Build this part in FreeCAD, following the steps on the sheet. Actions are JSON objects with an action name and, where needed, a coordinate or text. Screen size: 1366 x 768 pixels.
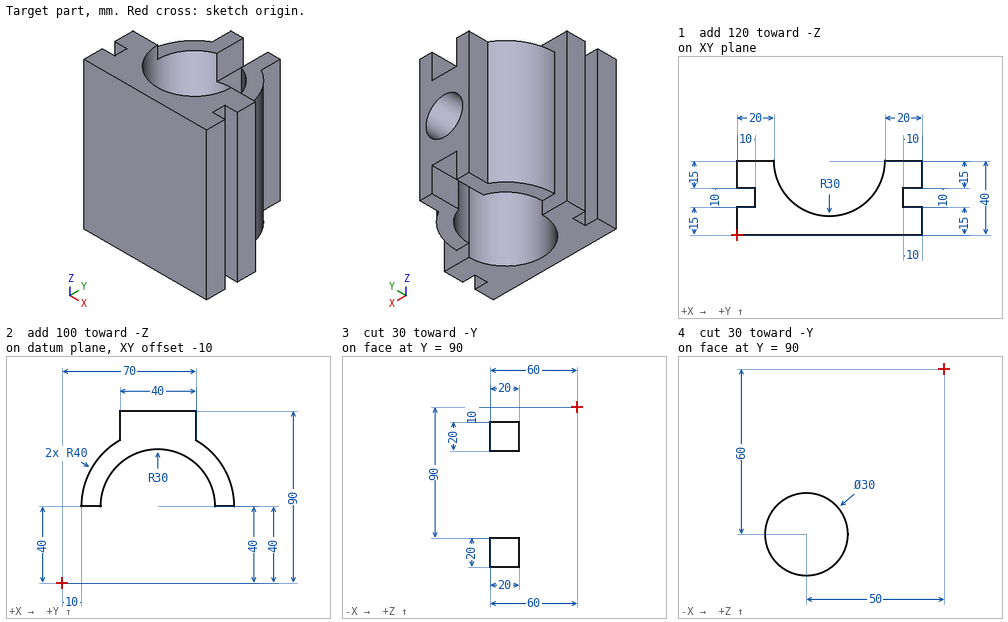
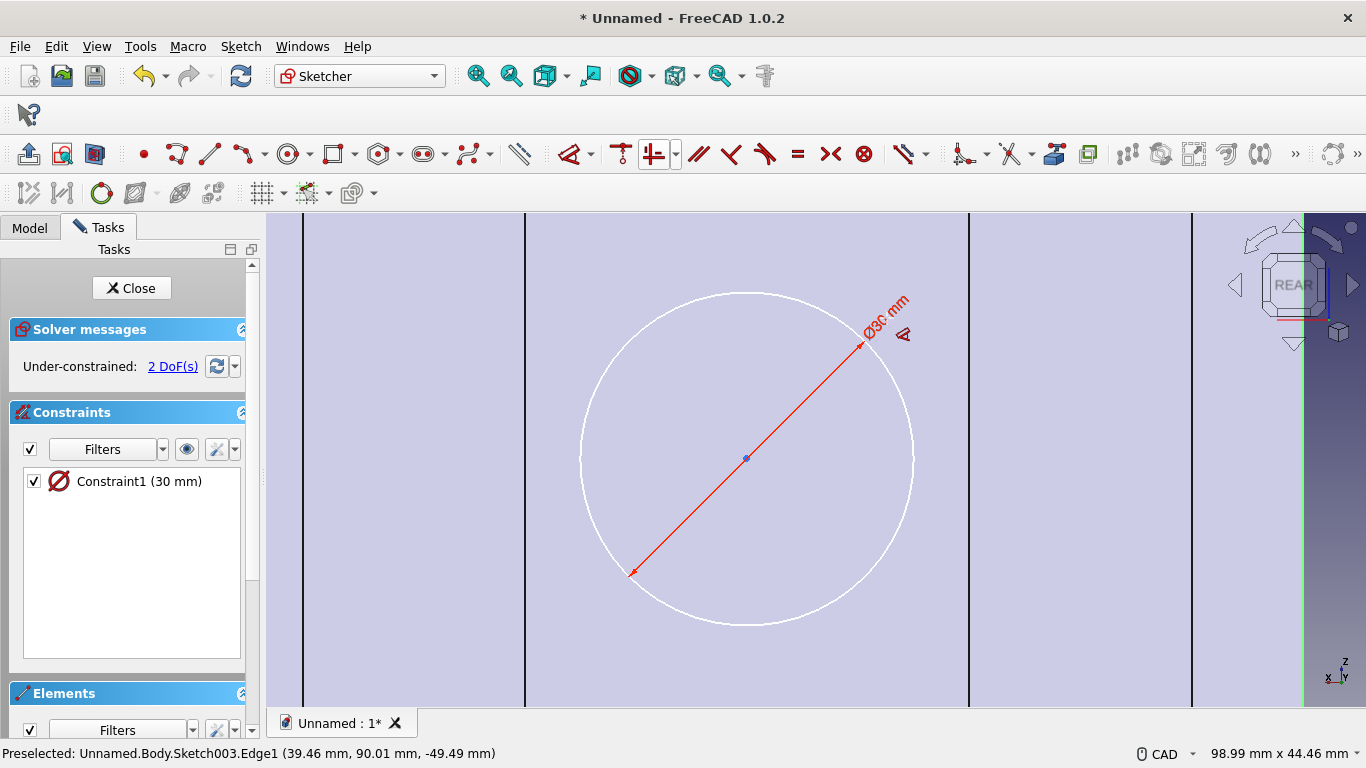
{"action": "left_click", "coordinate": [747, 459]}
{"action": "left_click", "coordinate": [974, 493]}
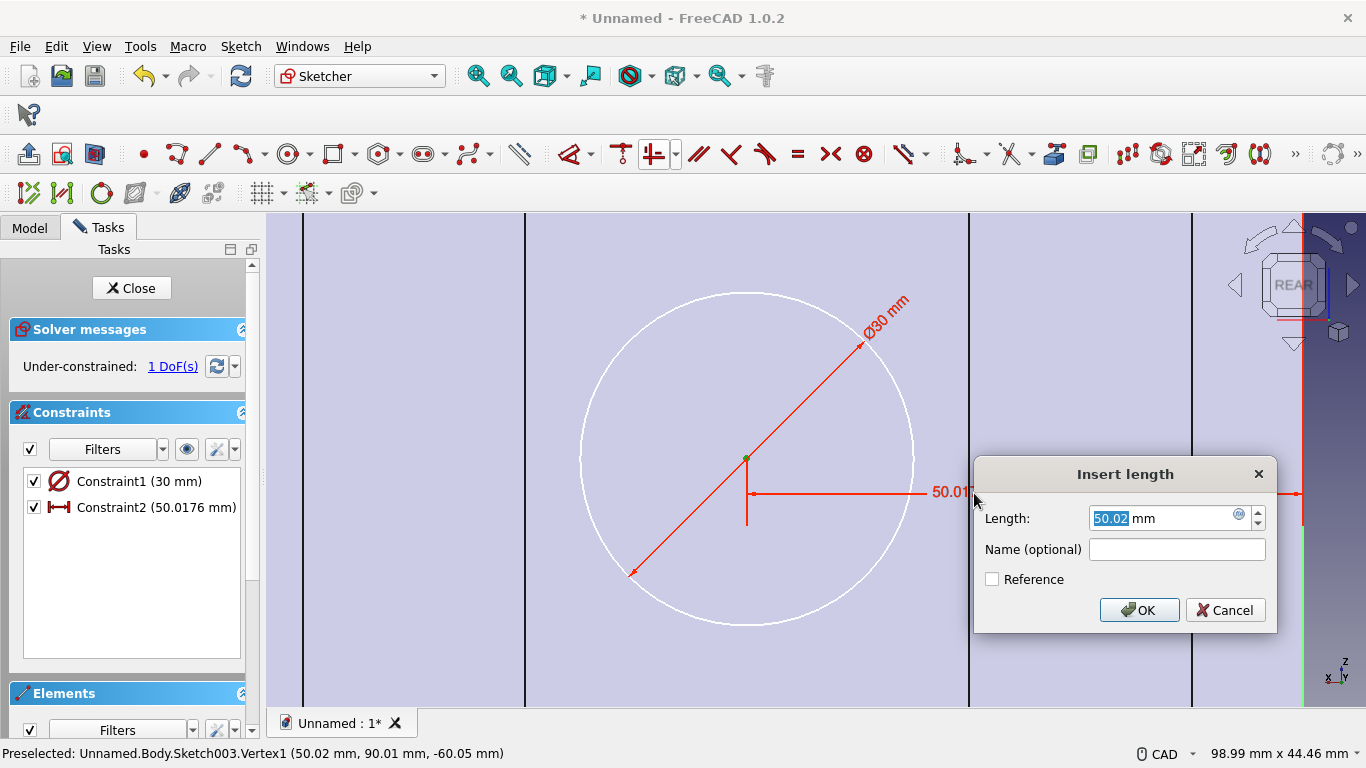
{"action": "type", "text": "50"}
{"action": "key", "text": "Return"}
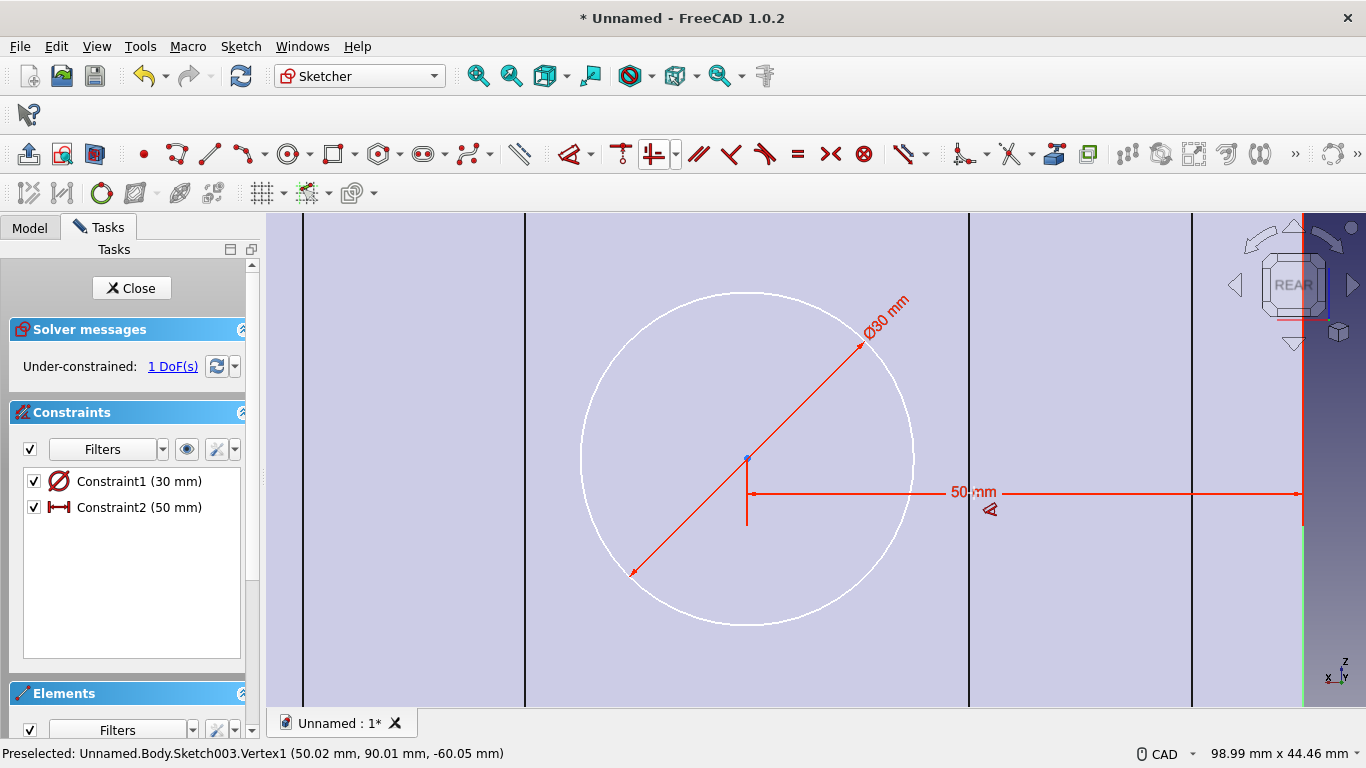
{"action": "left_click", "coordinate": [747, 459]}
{"action": "left_click", "coordinate": [713, 350]}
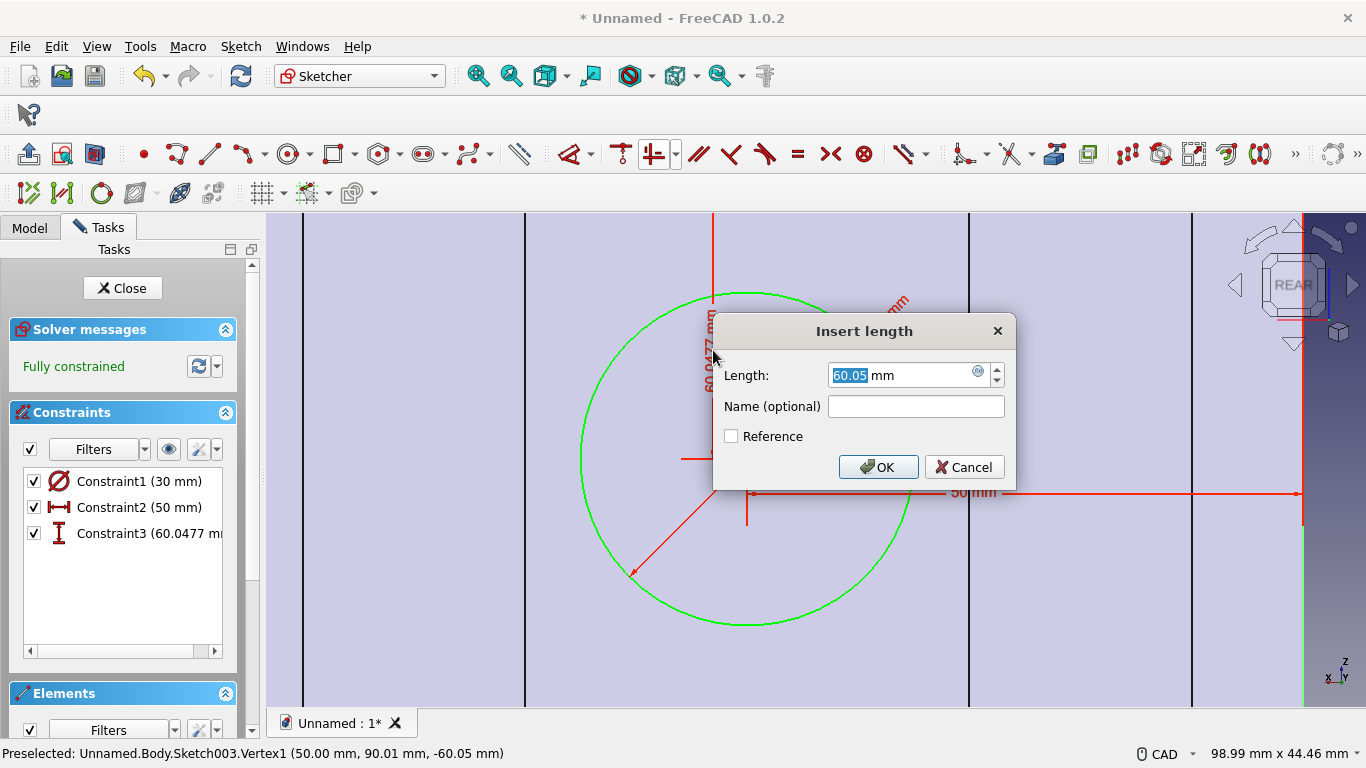
{"action": "type", "text": "60"}
{"action": "key", "text": "Return"}
{"action": "key", "text": "Escape"}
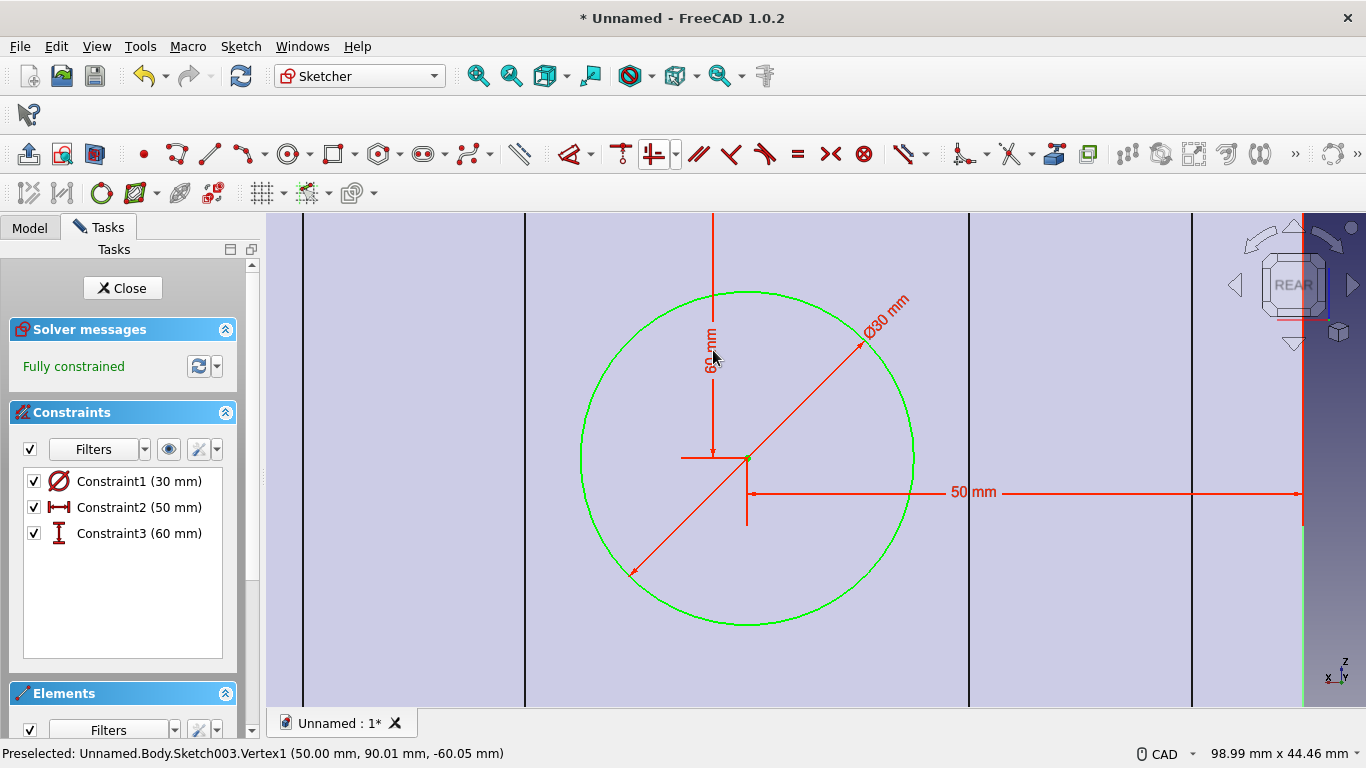
{"action": "left_click", "coordinate": [123, 288]}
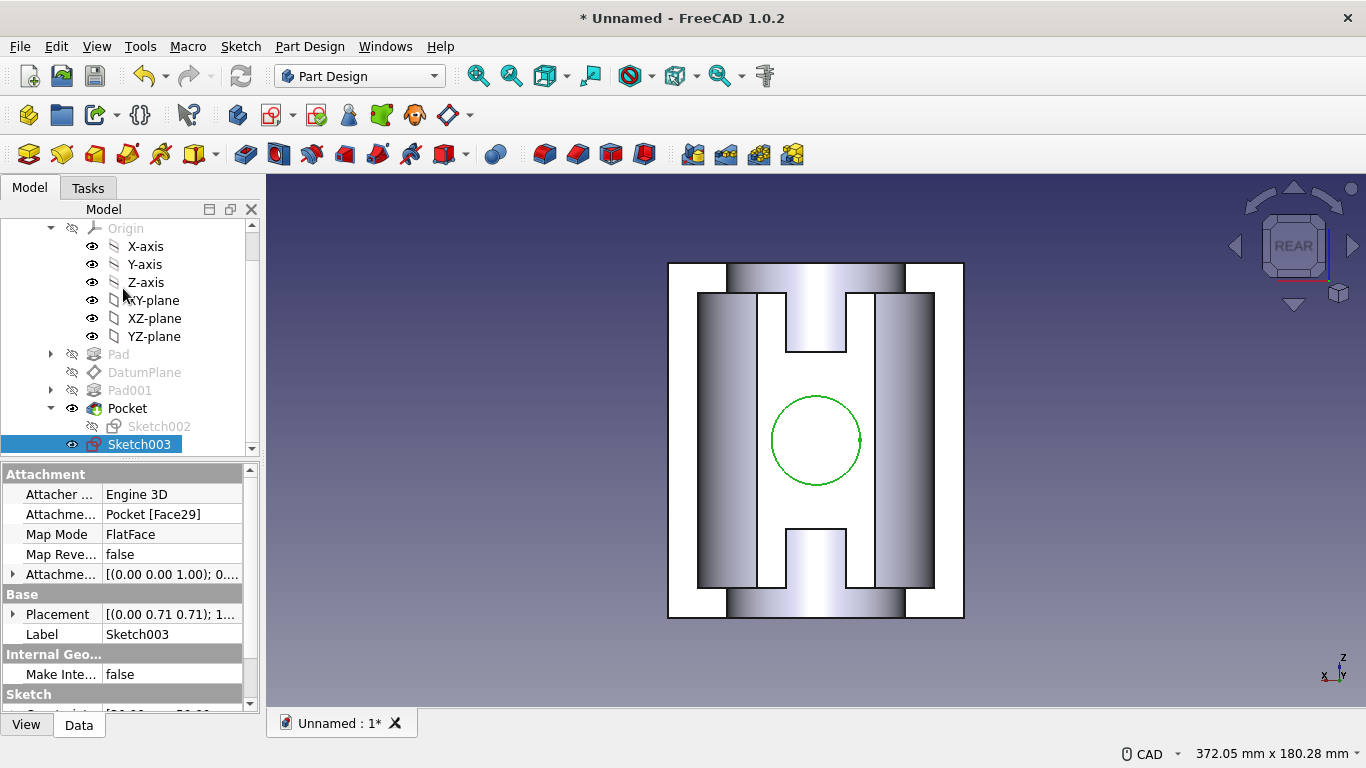
{"action": "left_click", "coordinate": [246, 154]}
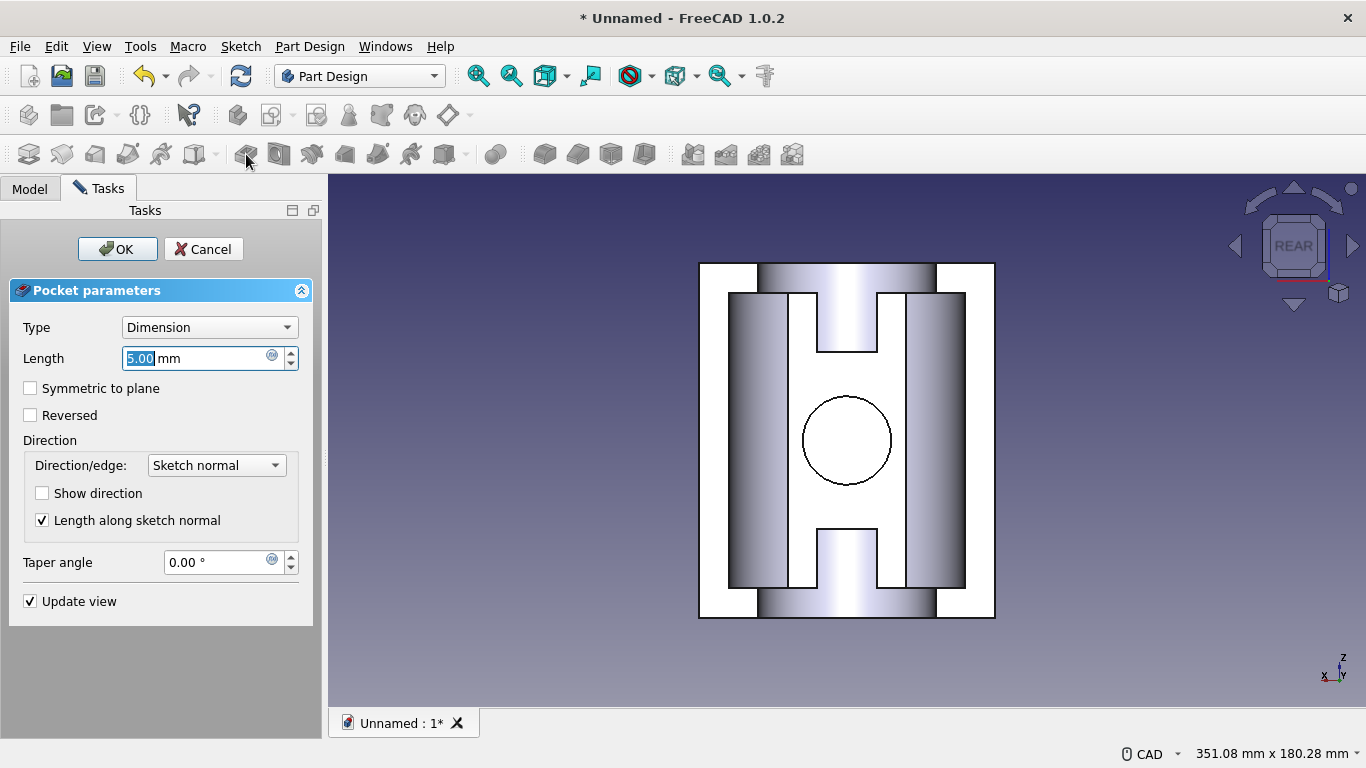
{"action": "type", "text": "30"}
{"action": "key", "text": "Tab"}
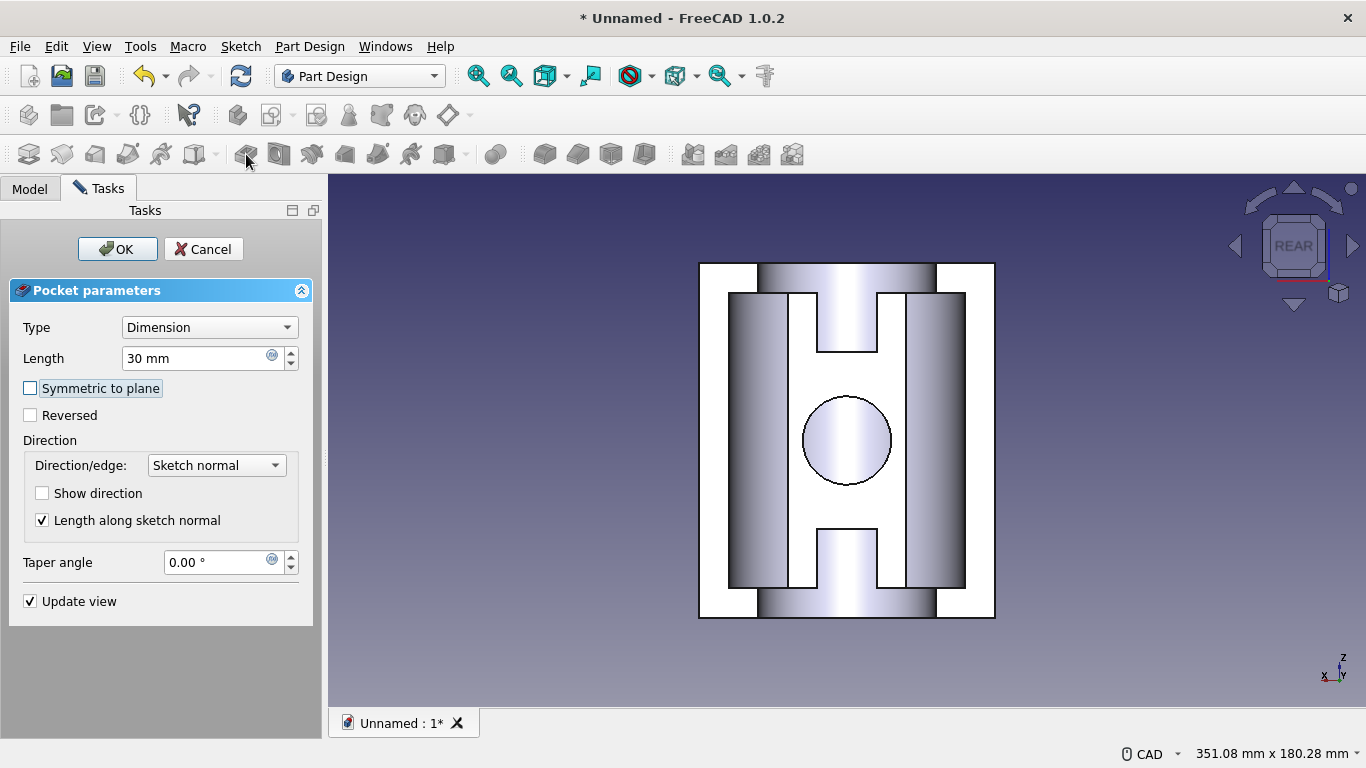
{"action": "left_click", "coordinate": [118, 249]}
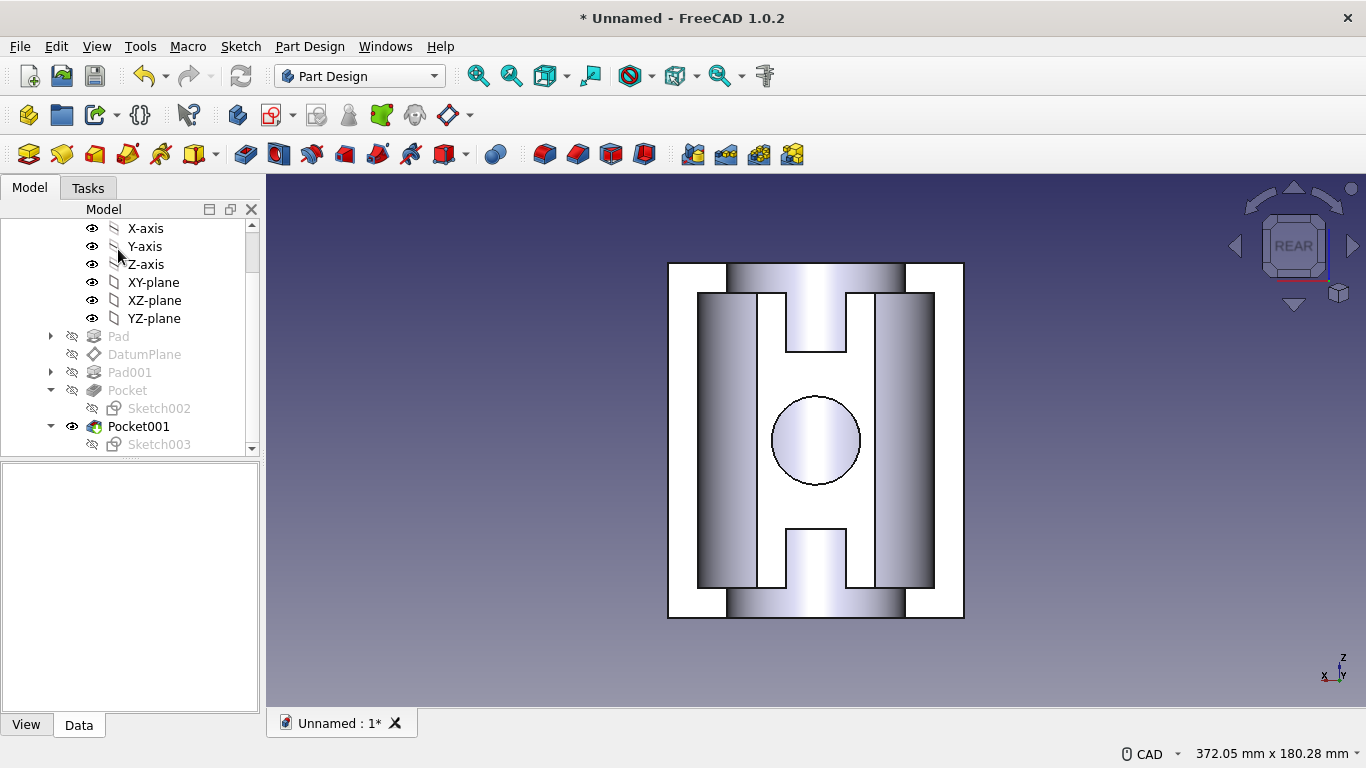
{"action": "key", "text": "0"}